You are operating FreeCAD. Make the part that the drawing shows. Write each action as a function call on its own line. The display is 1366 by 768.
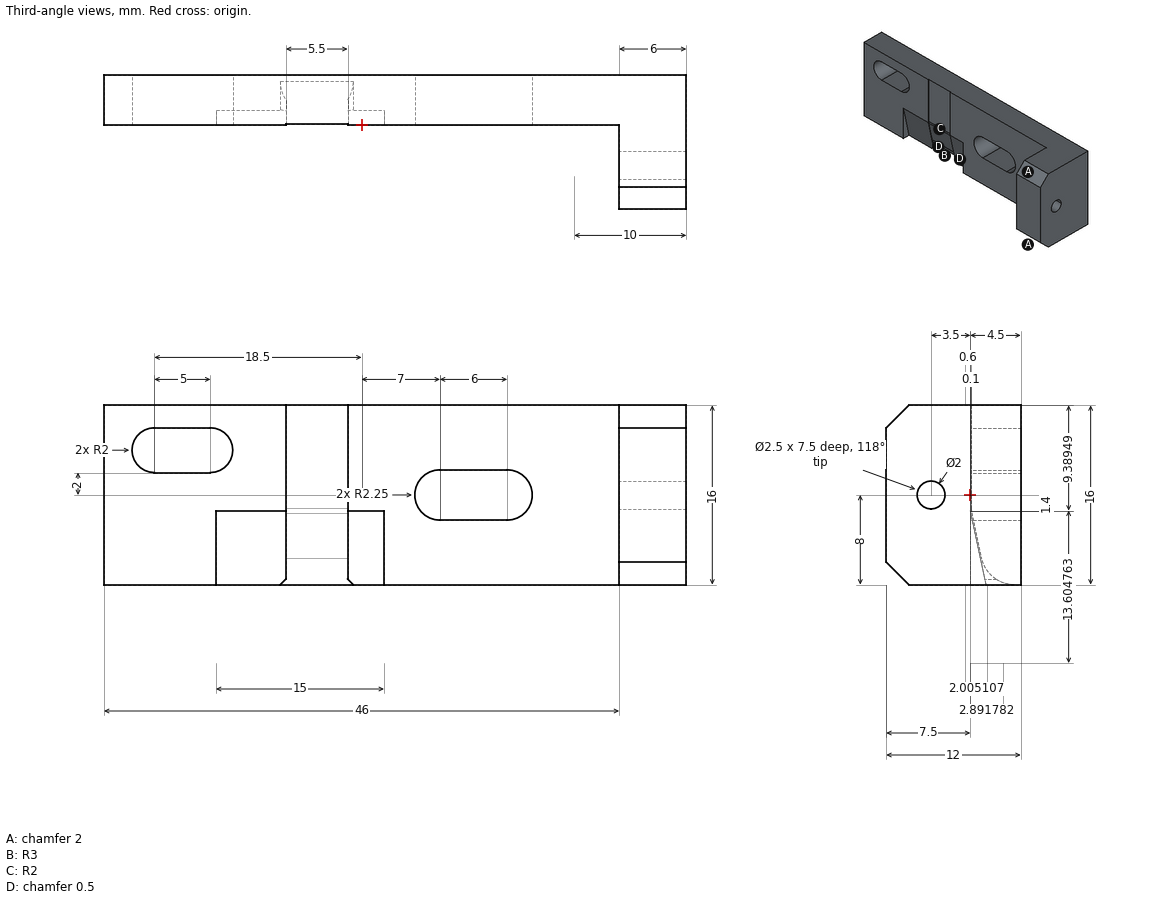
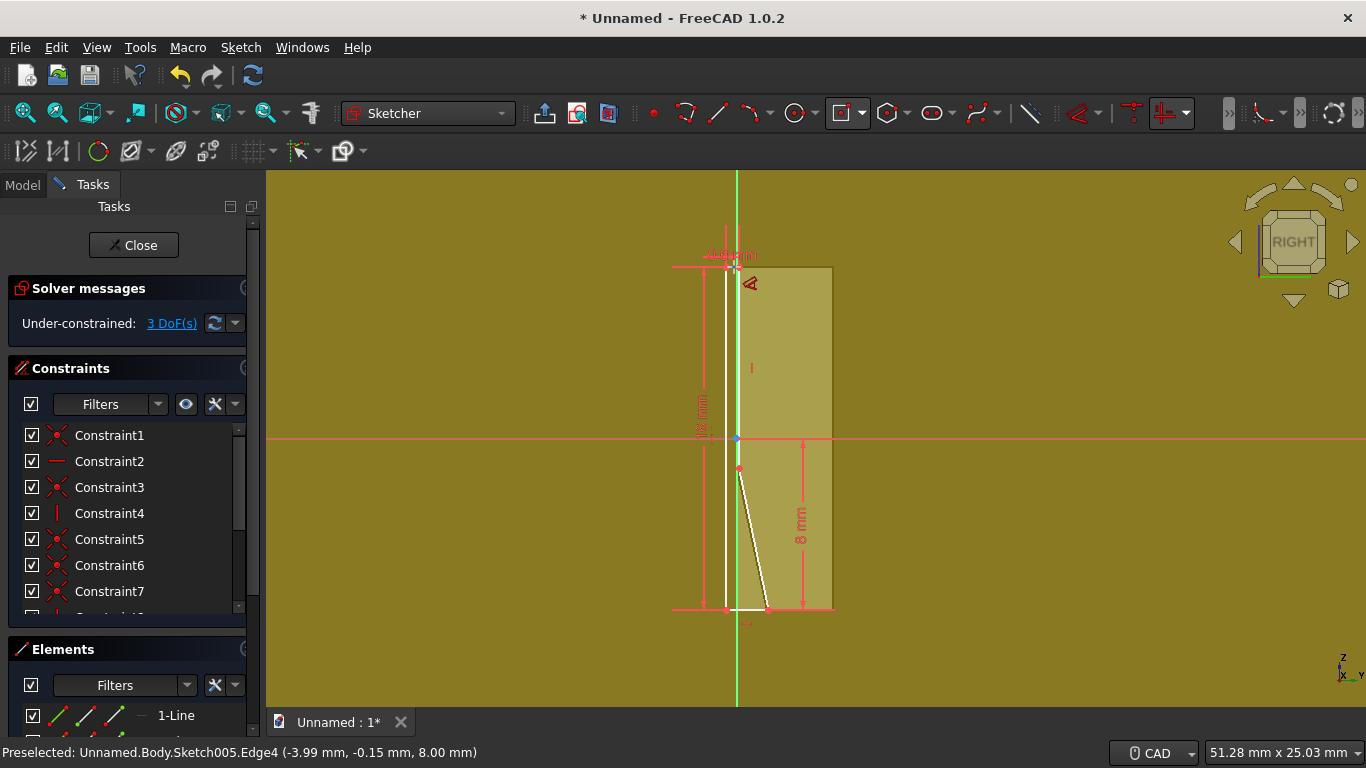
scroll(739, 469, up, 15)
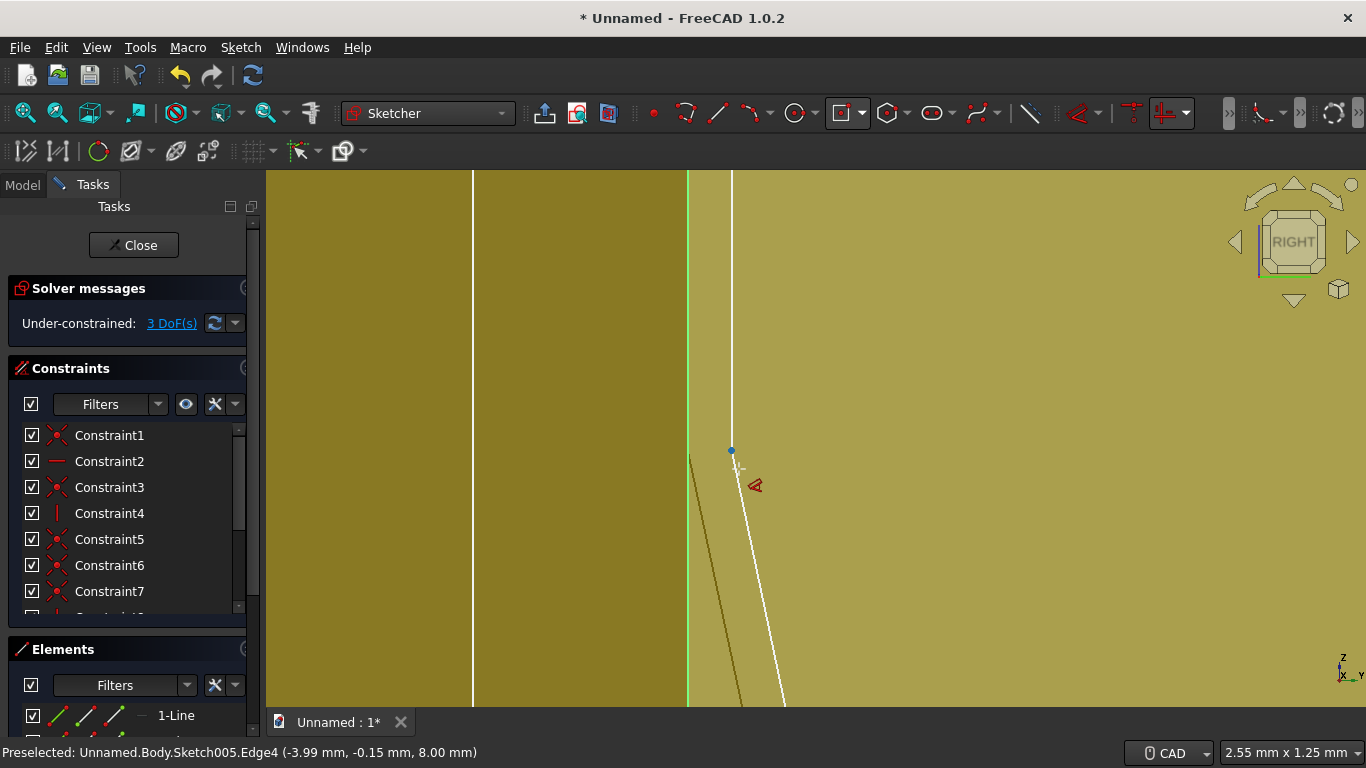
click(732, 451)
click(710, 485)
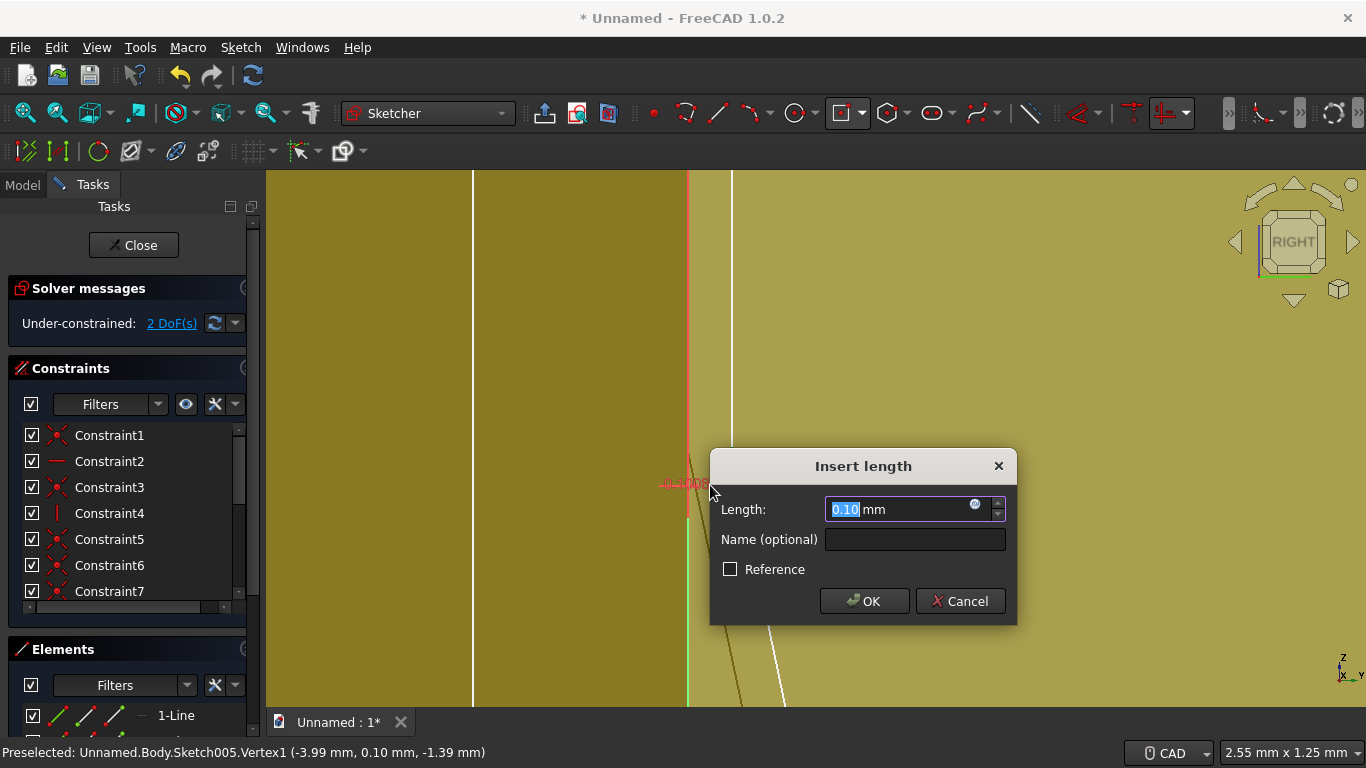
text(0.1)
key(Return)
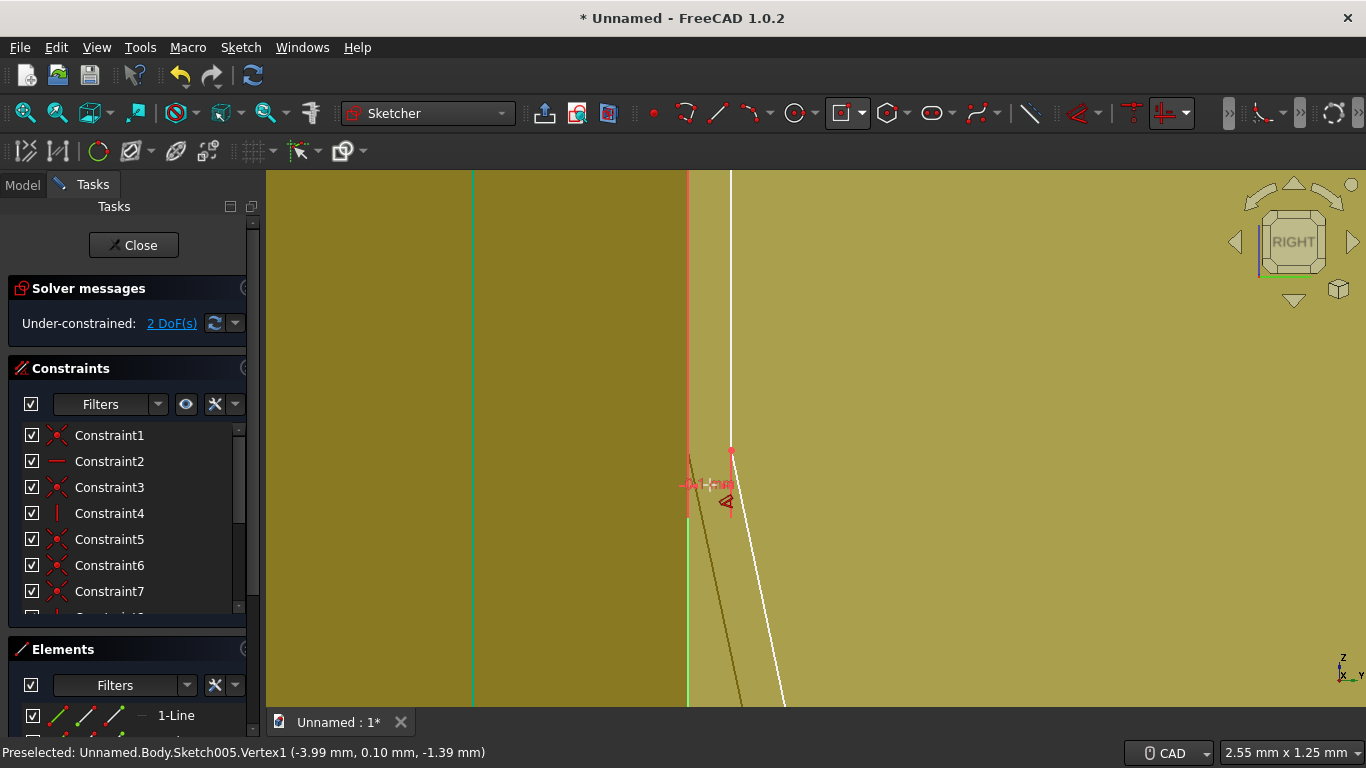
scroll(739, 469, down, 15)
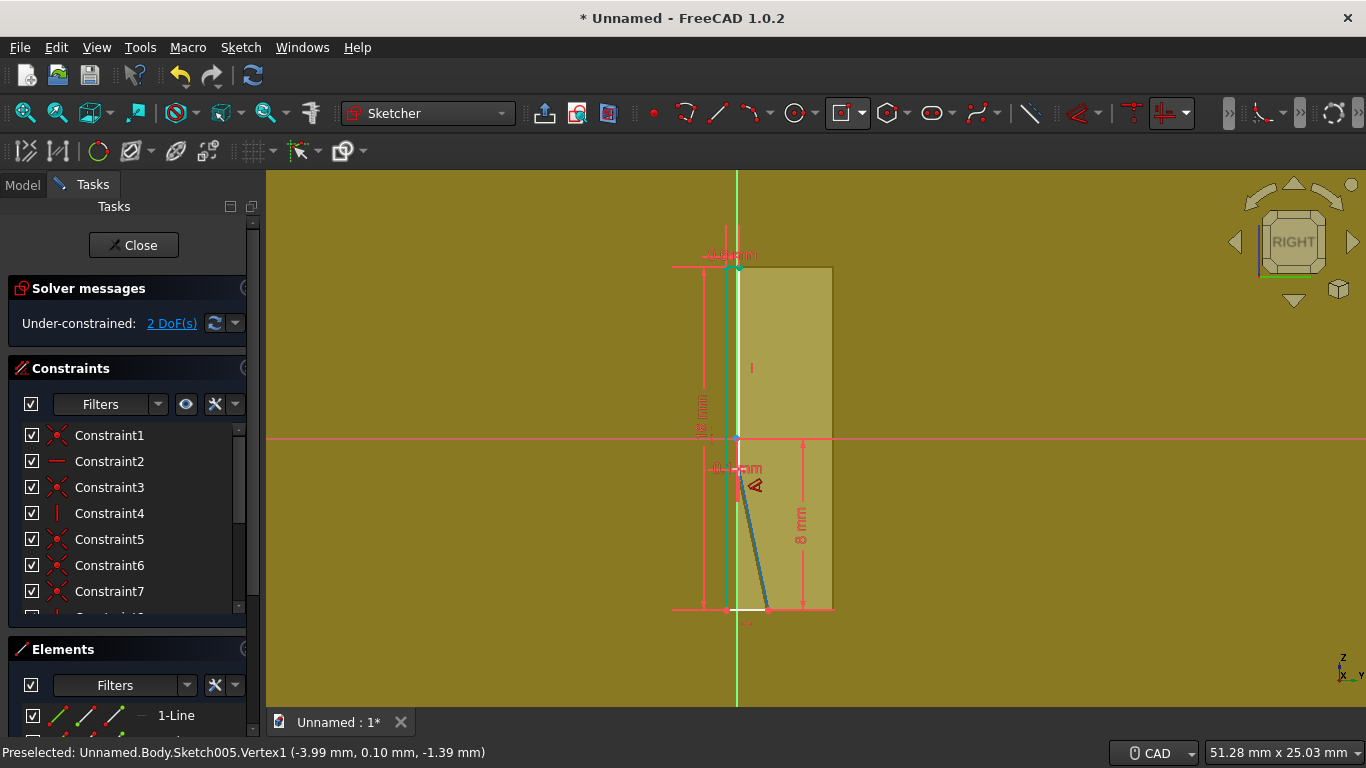
scroll(739, 328, up, 10)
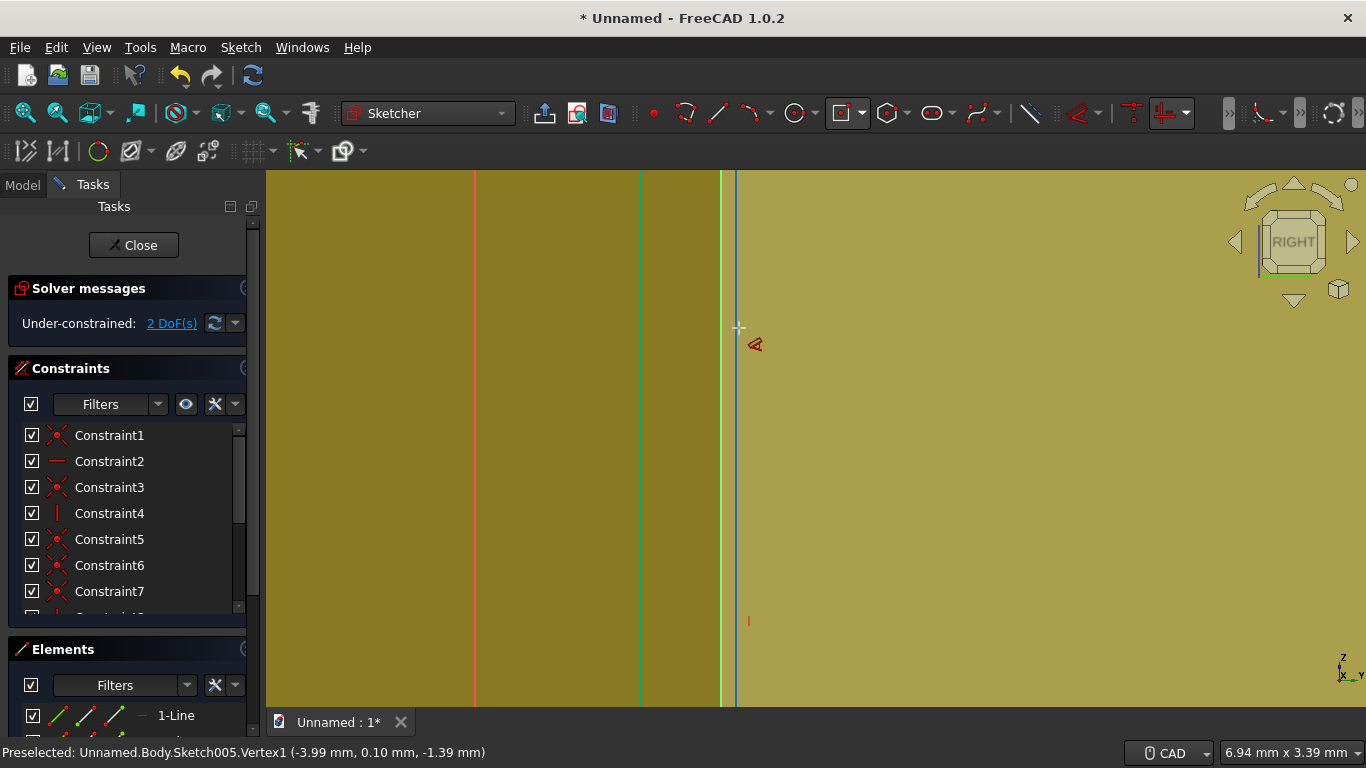
click(736, 323)
click(702, 438)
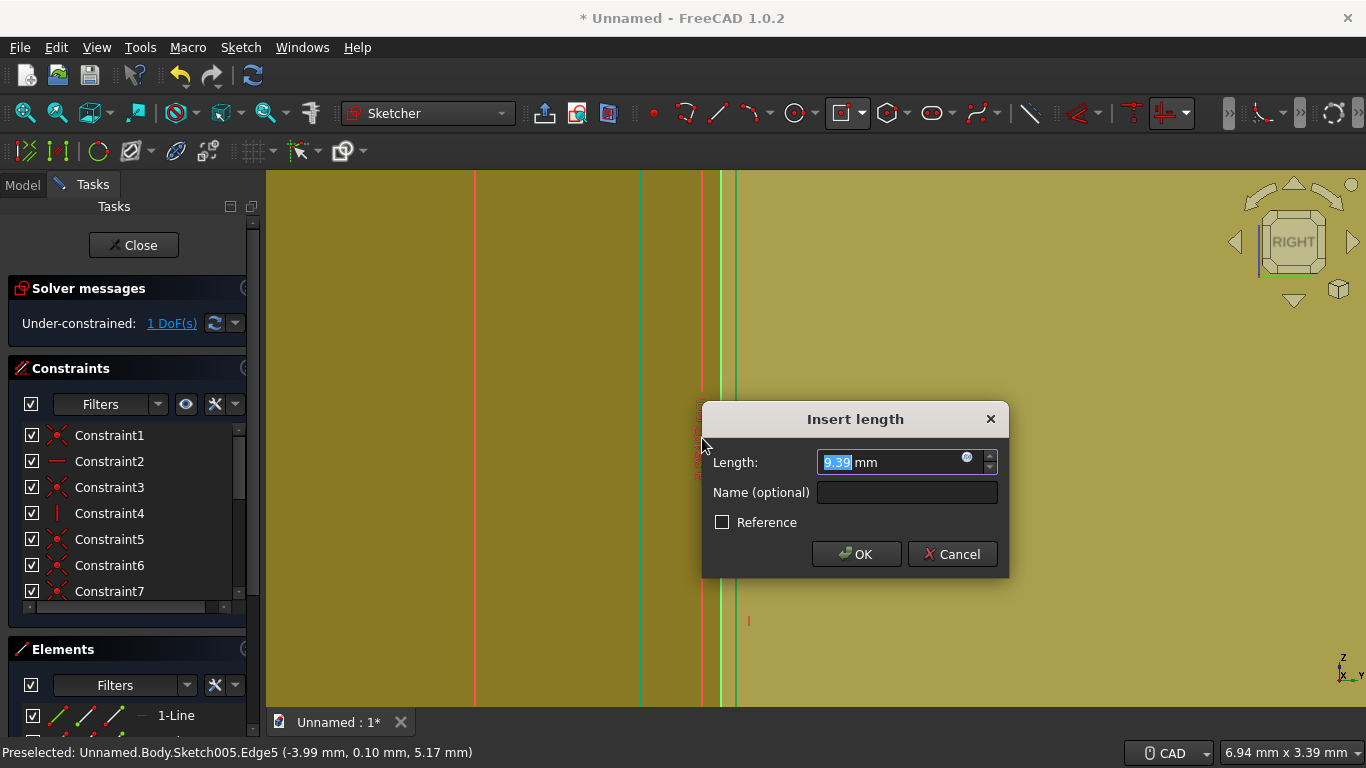
text(9.38949)
key(Return)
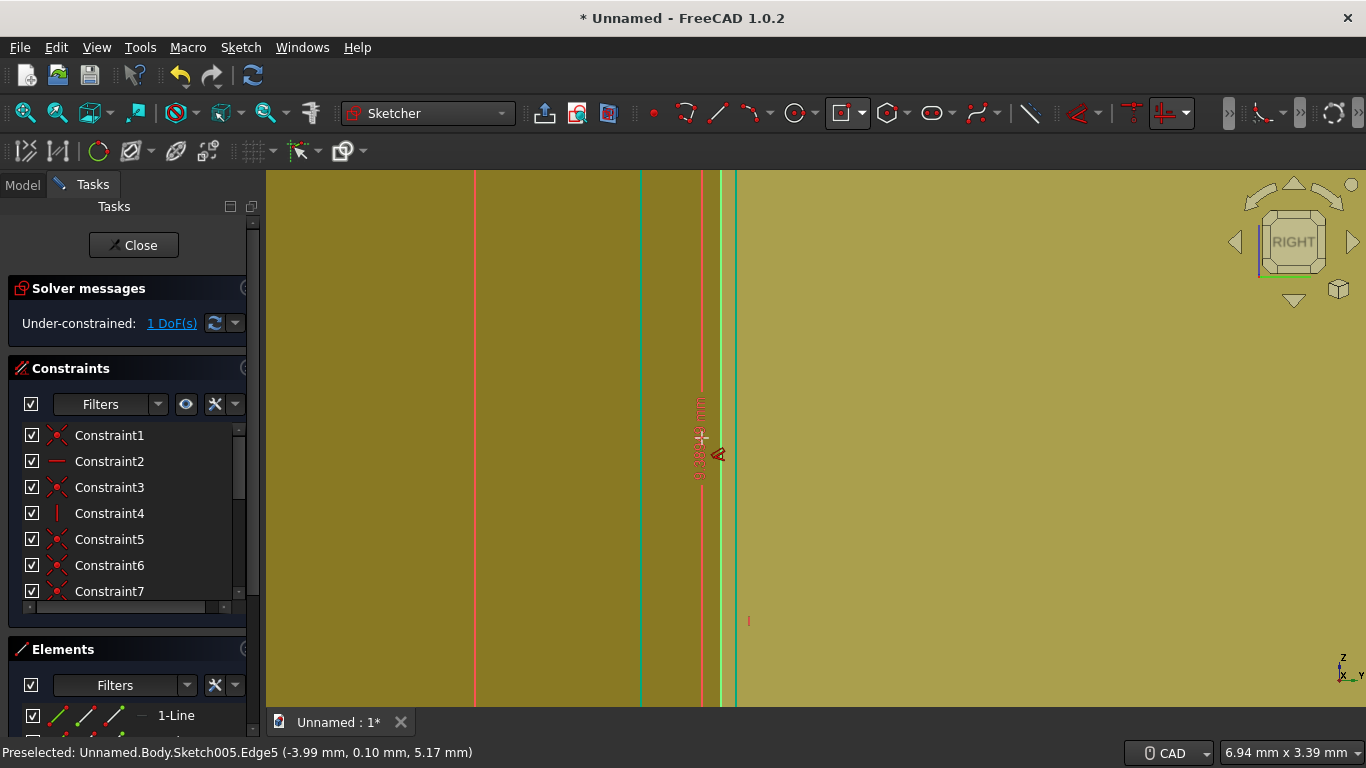
scroll(739, 328, down, 10)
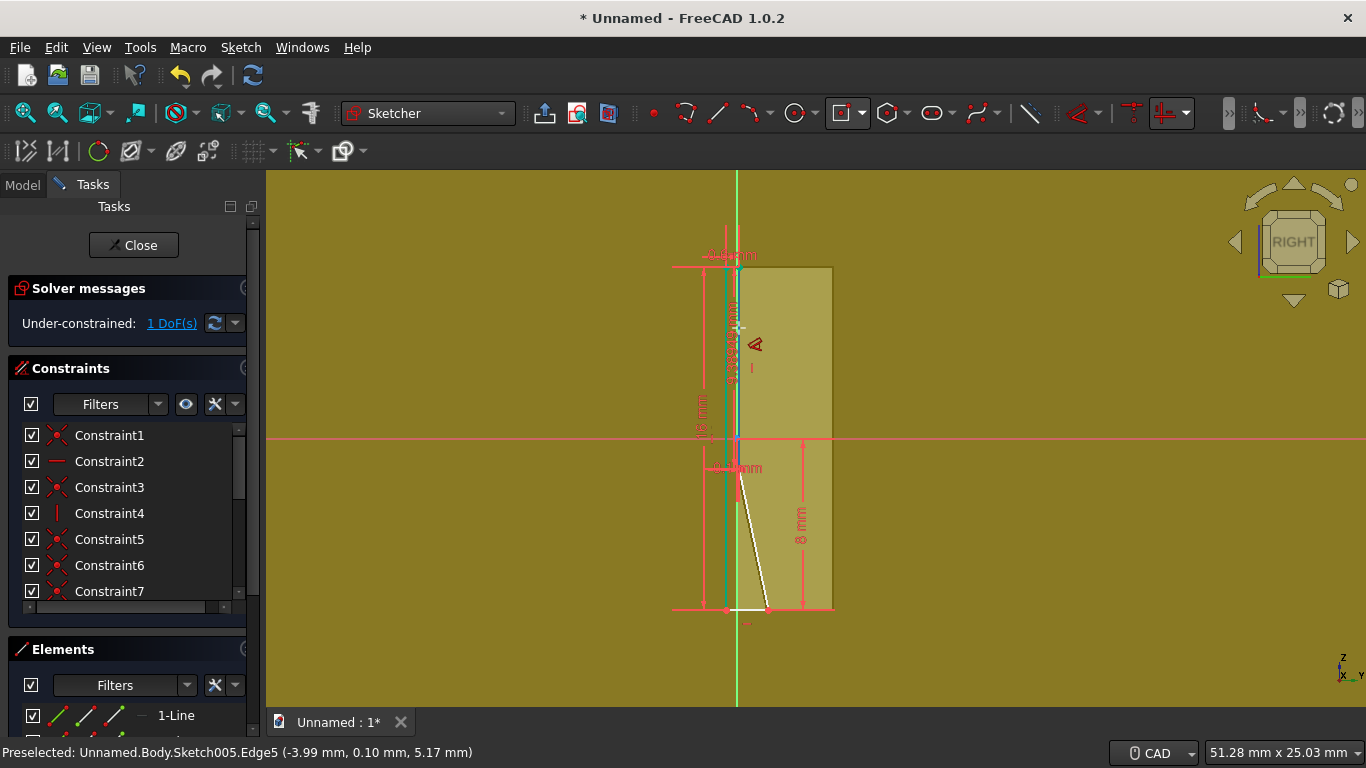
click(756, 610)
click(757, 644)